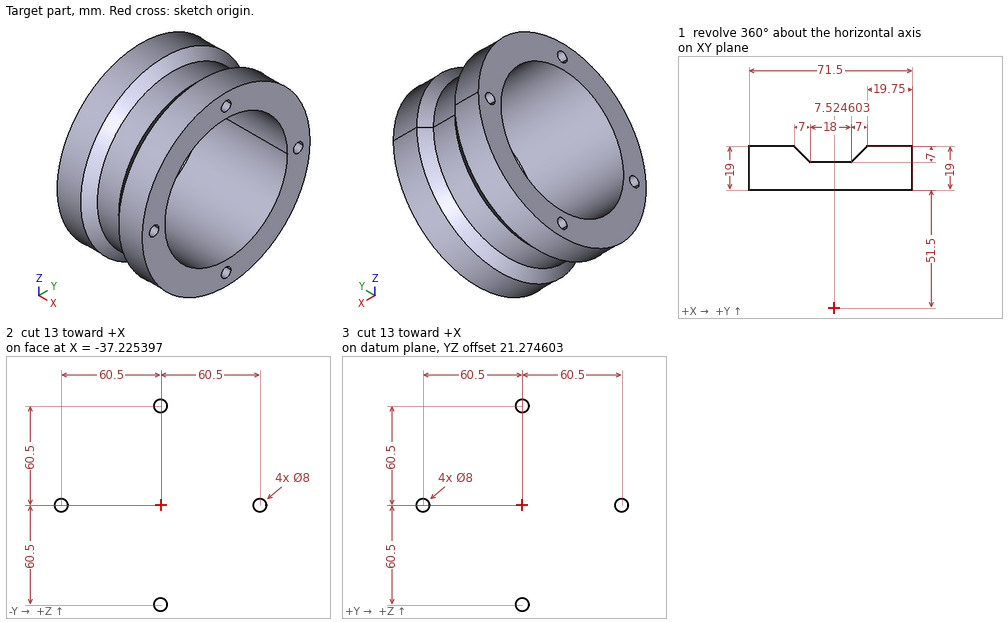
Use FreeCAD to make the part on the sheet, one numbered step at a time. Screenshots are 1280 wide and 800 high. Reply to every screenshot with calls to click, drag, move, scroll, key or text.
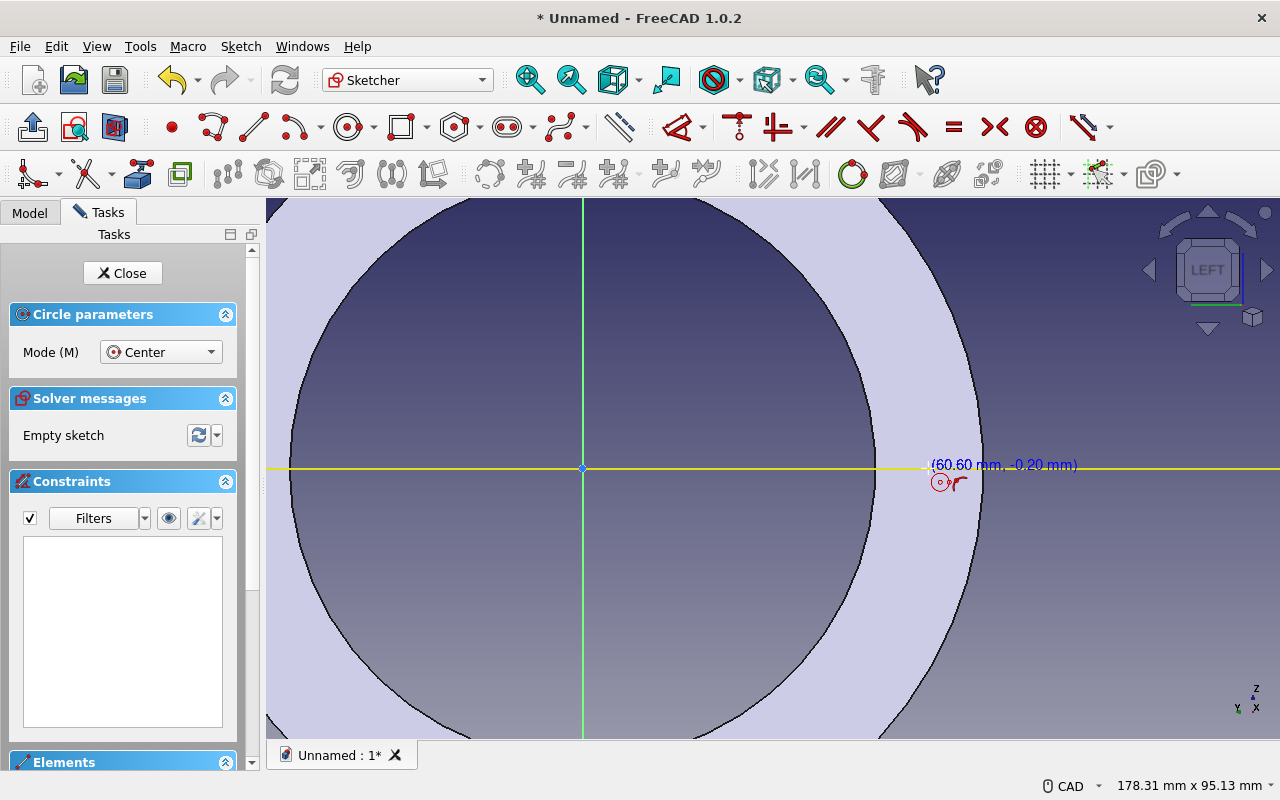
click(927, 468)
move(943, 452)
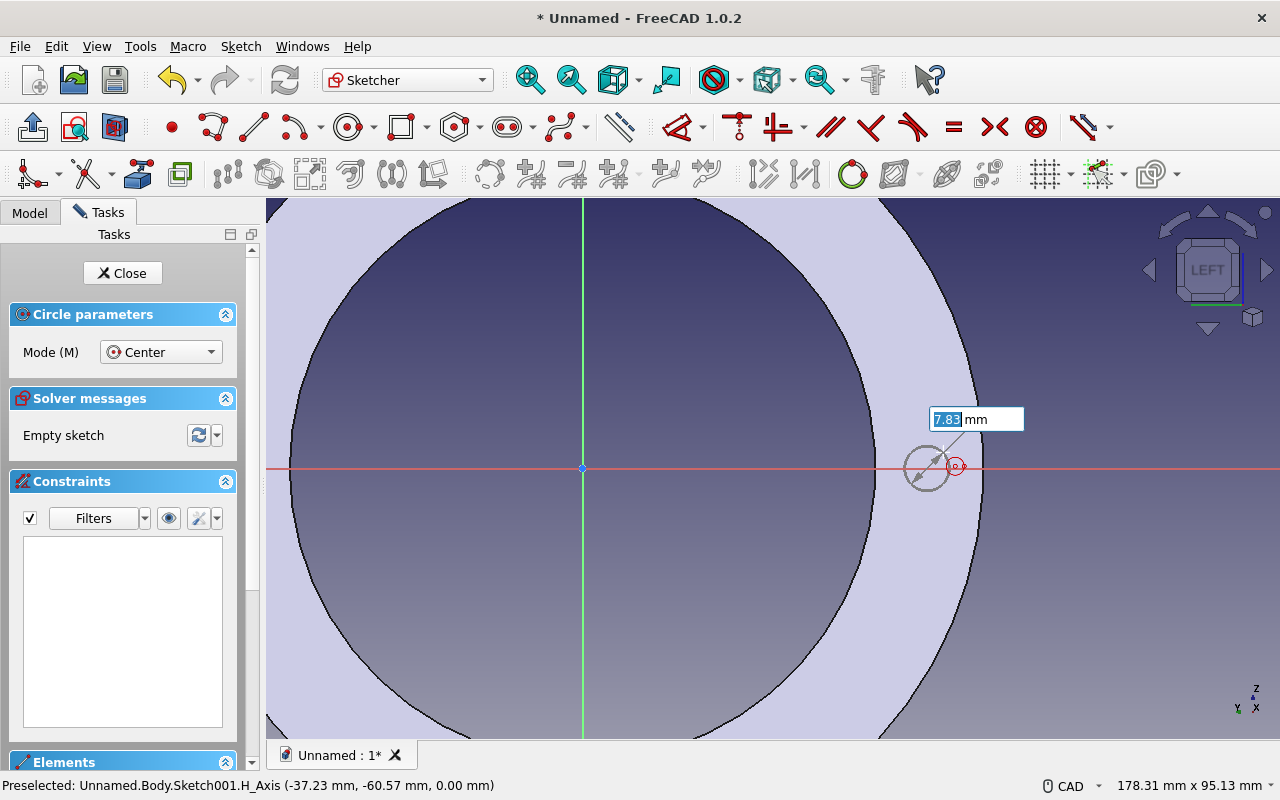
text(8)
key(Return)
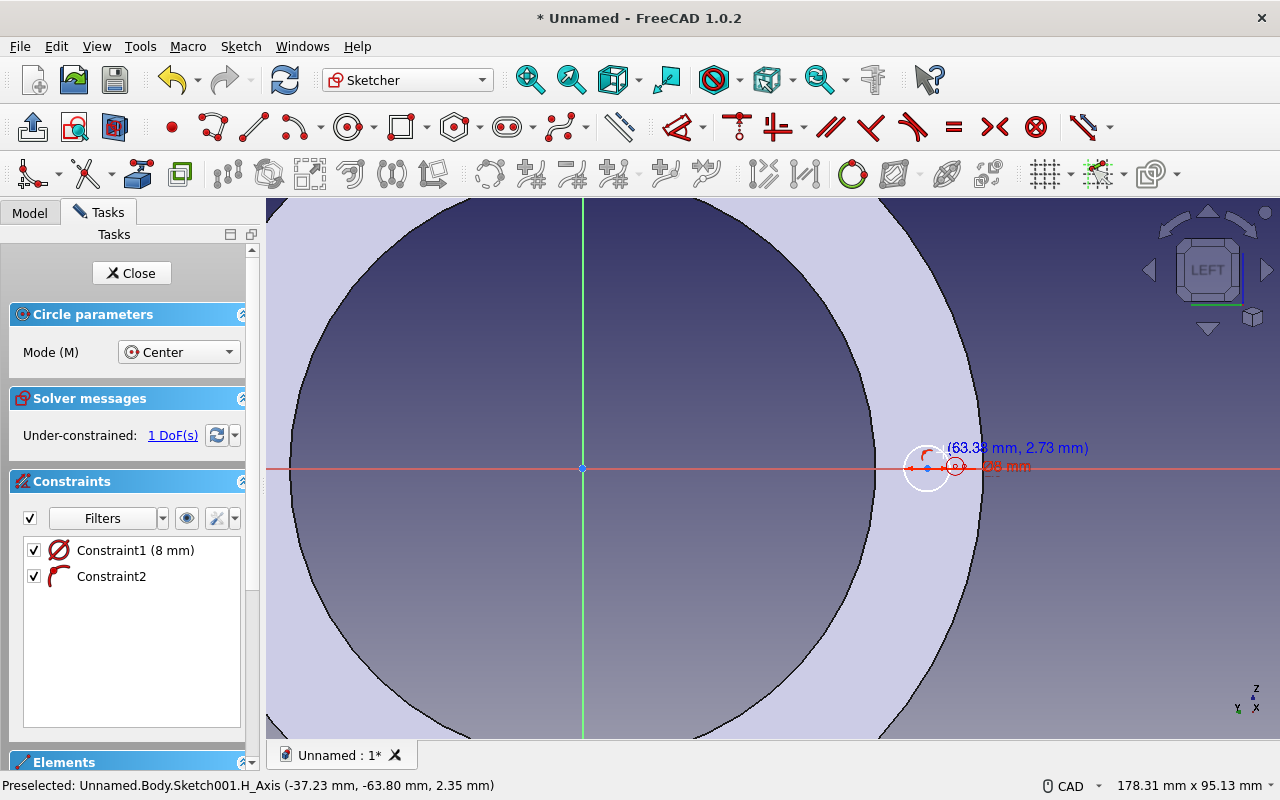
scroll(804, 469, down, 4)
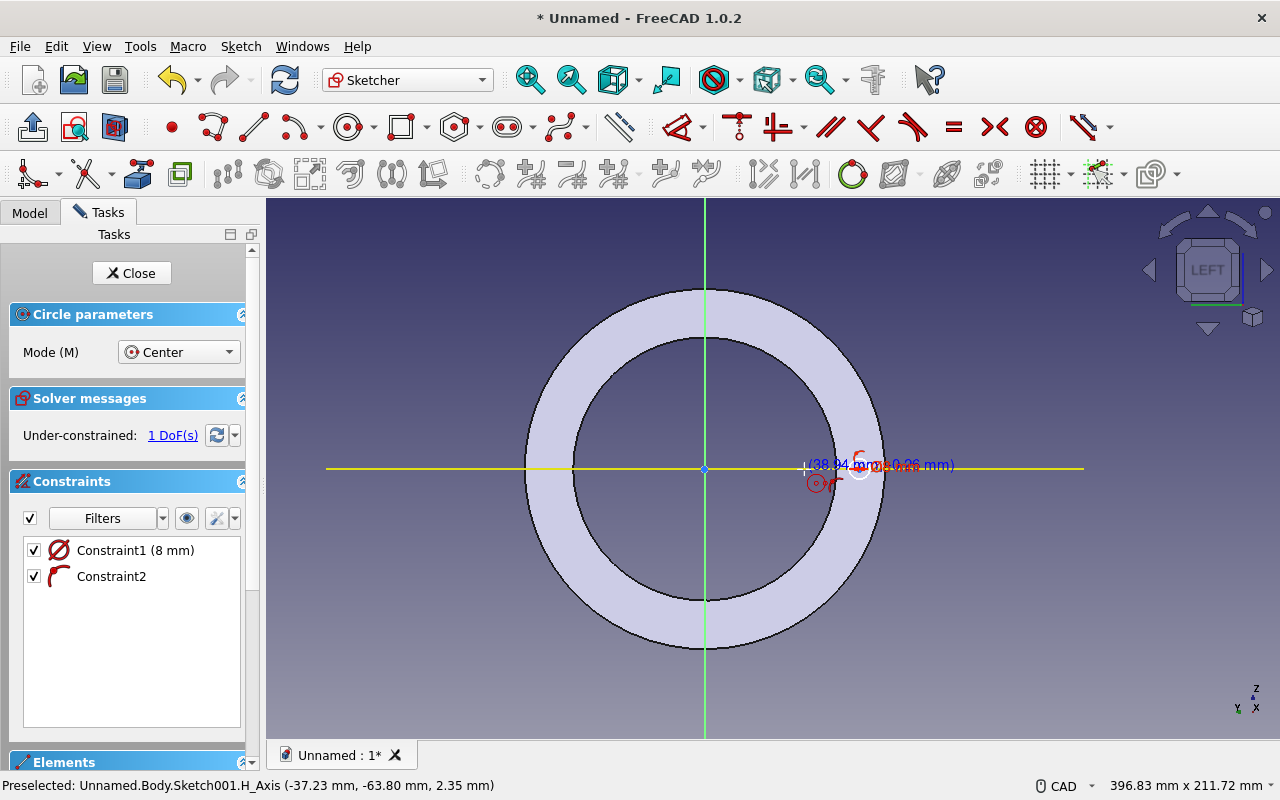
scroll(705, 624, up, 4)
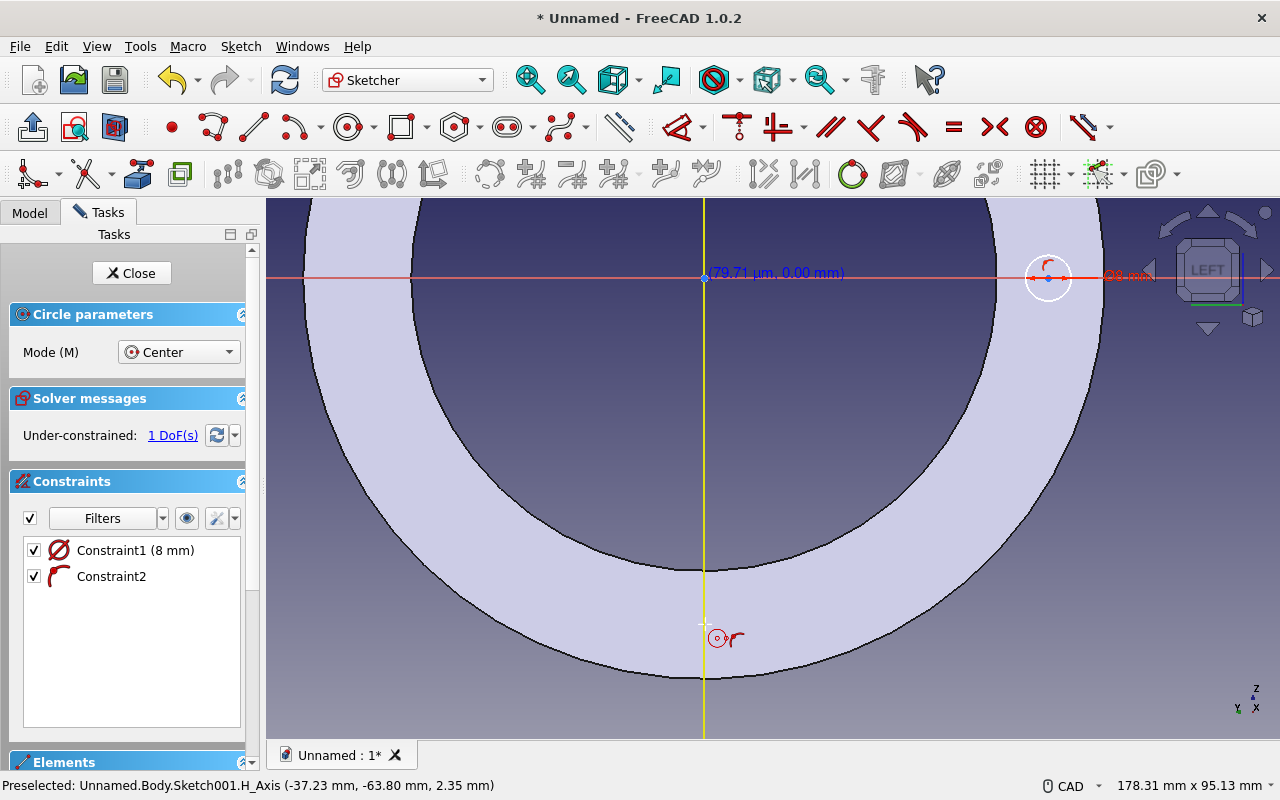
click(704, 622)
move(720, 606)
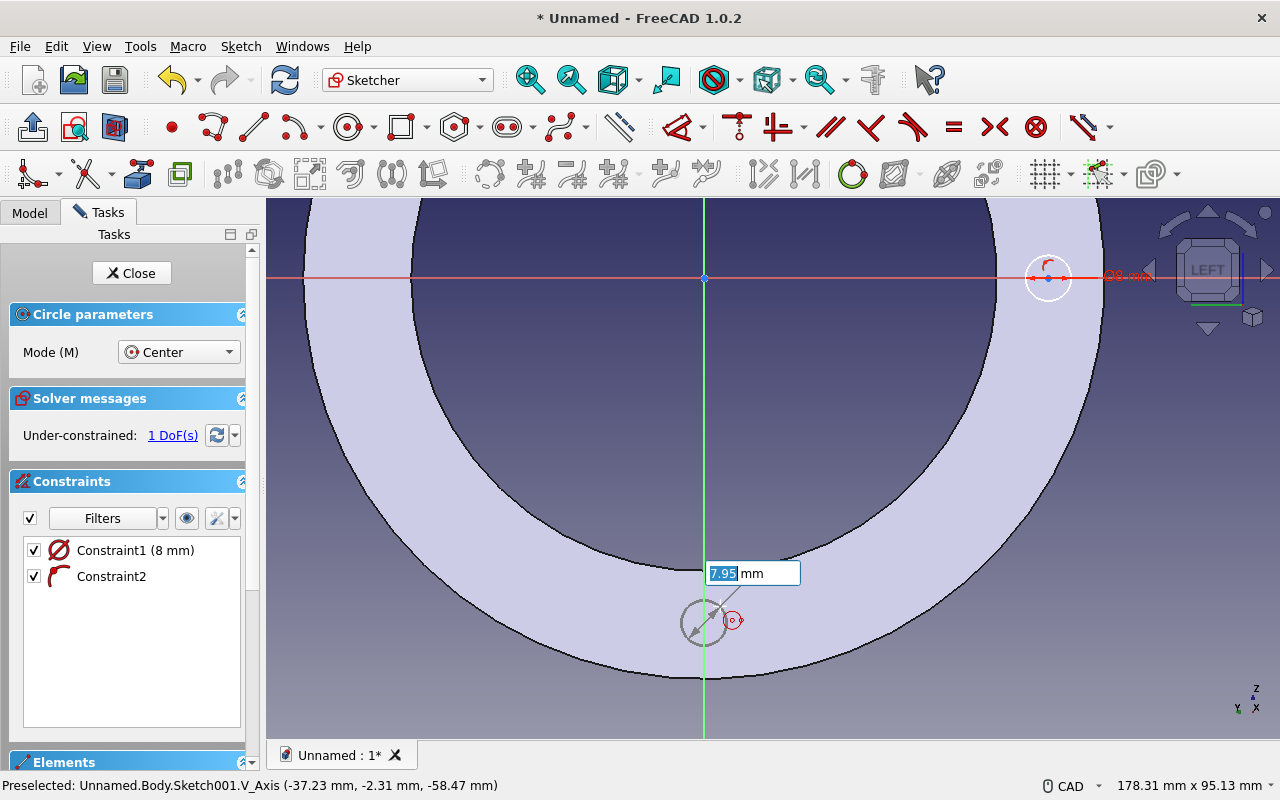
text(8)
key(Return)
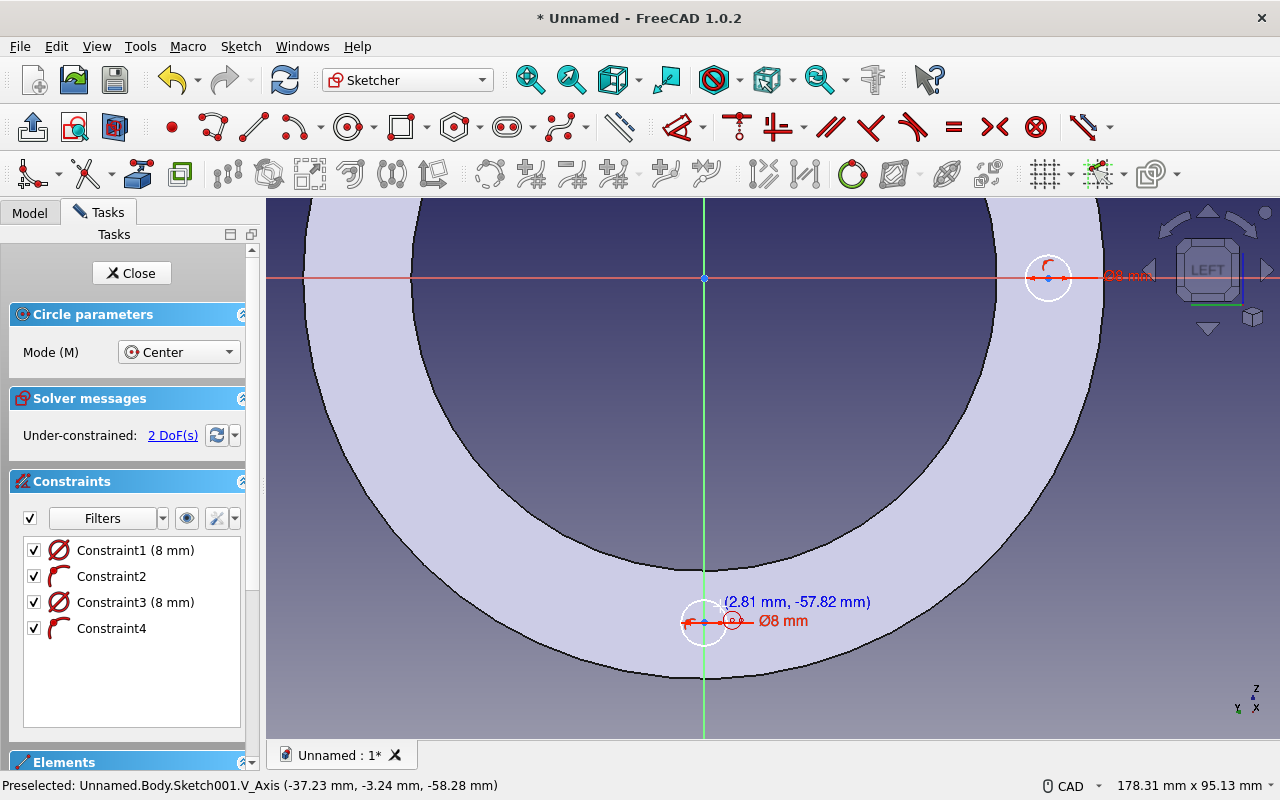
click(360, 278)
move(376, 262)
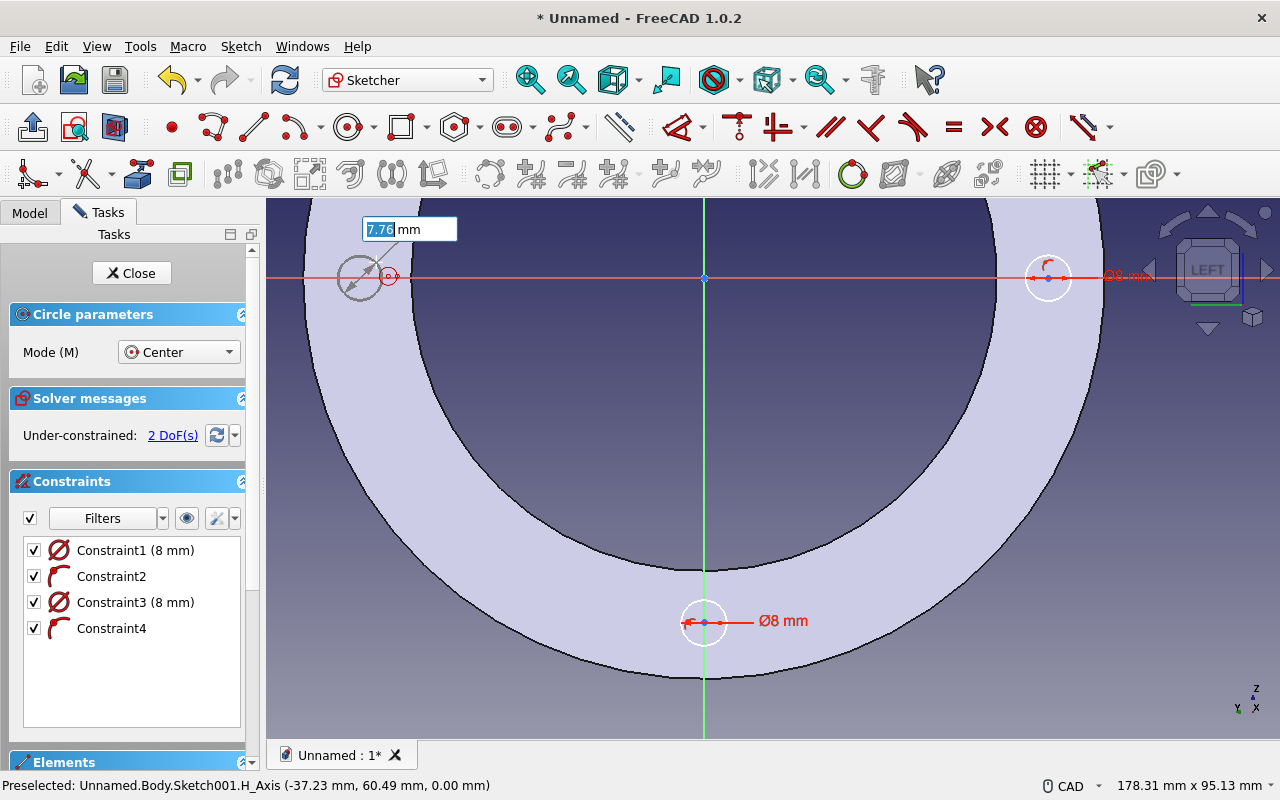
text(8)
key(Return)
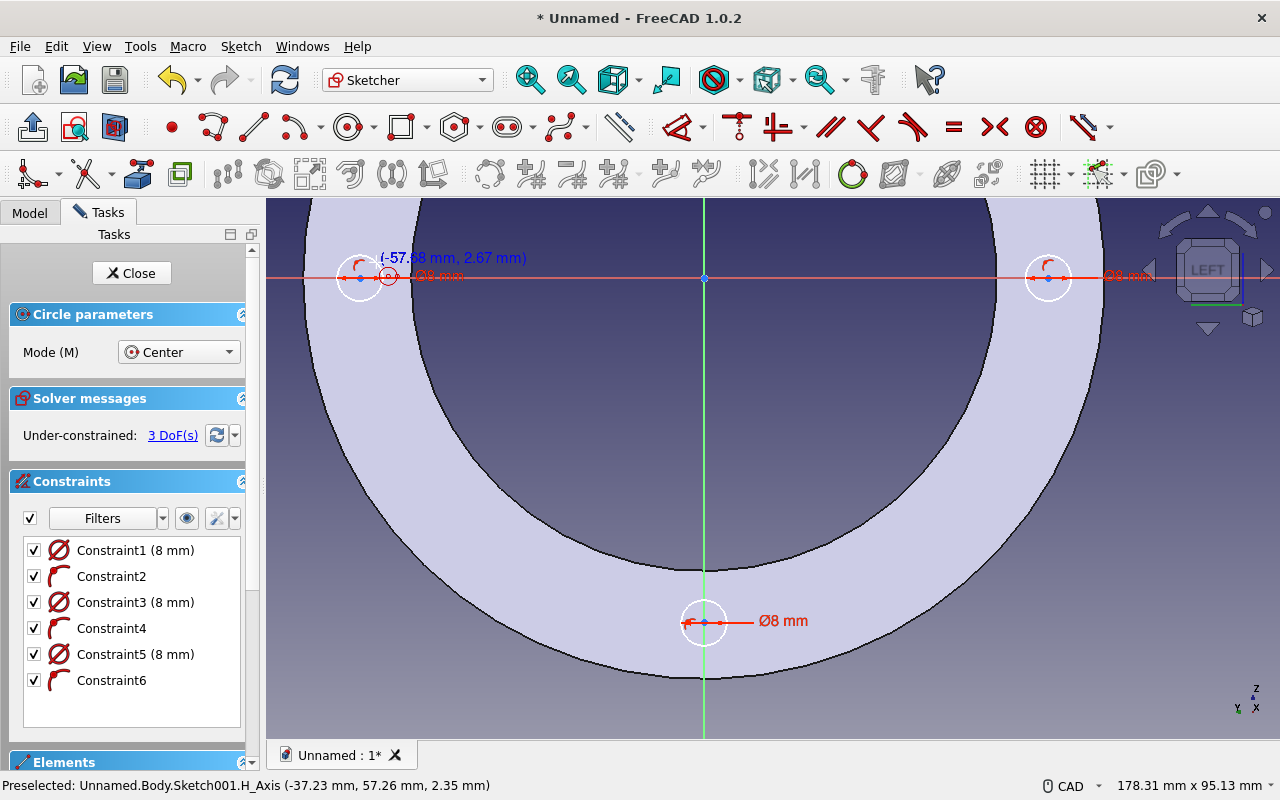
scroll(705, 624, down, 4)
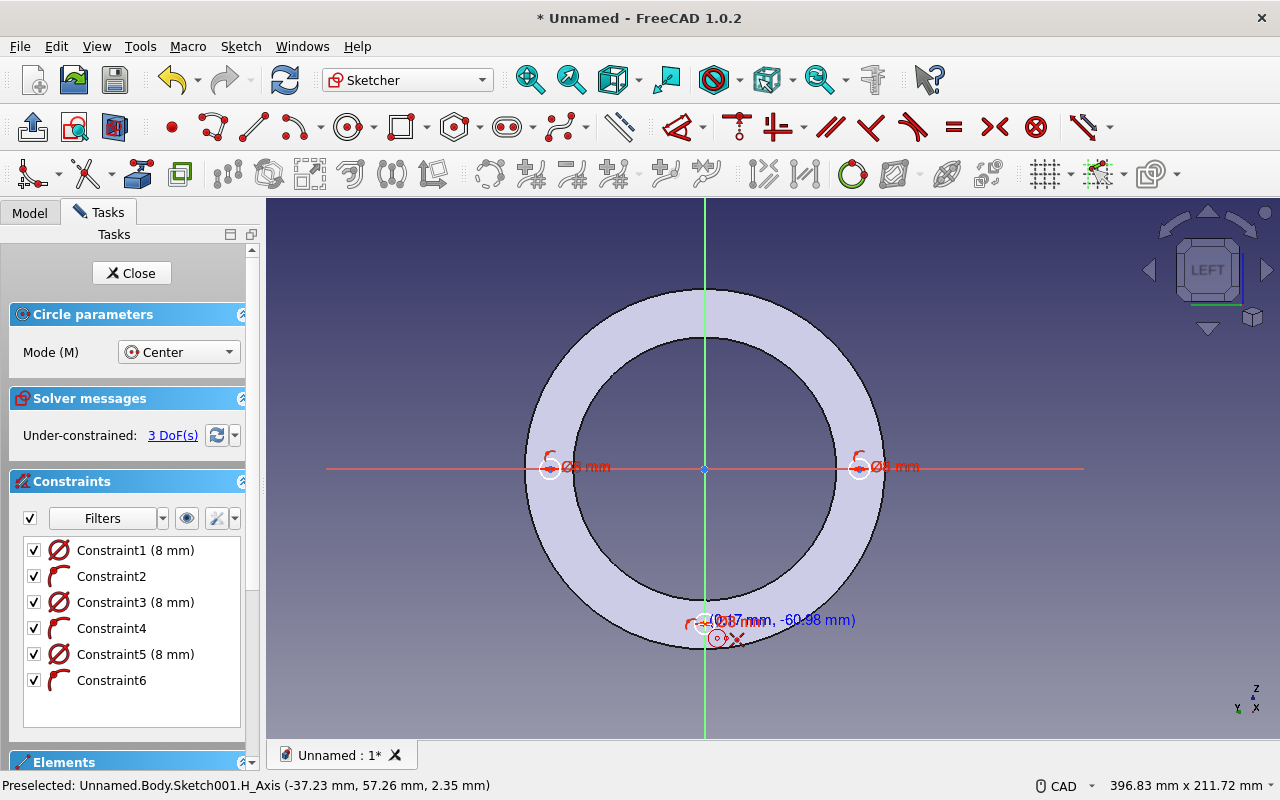
scroll(705, 314, up, 4)